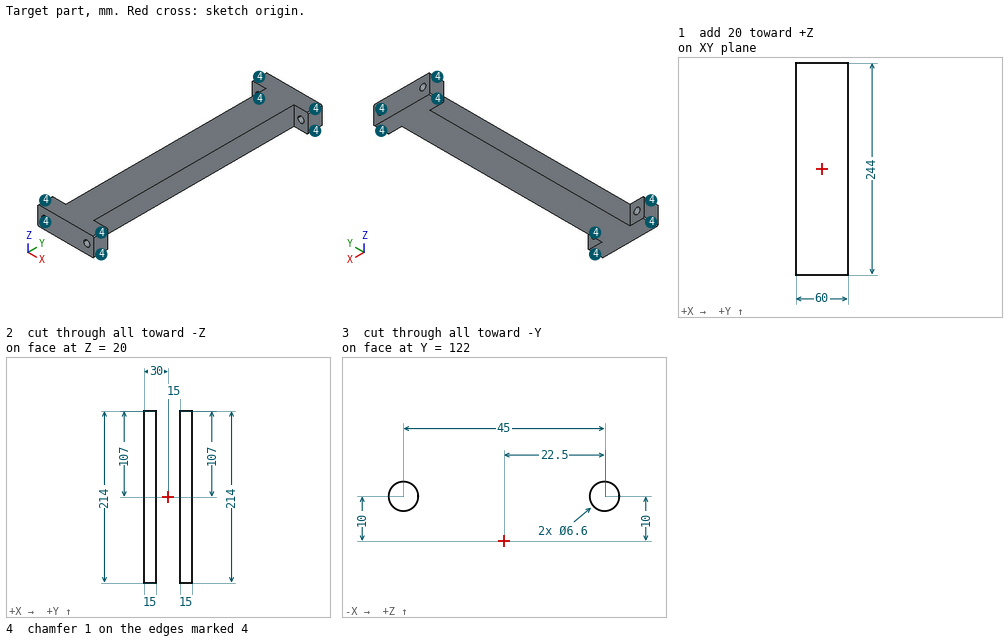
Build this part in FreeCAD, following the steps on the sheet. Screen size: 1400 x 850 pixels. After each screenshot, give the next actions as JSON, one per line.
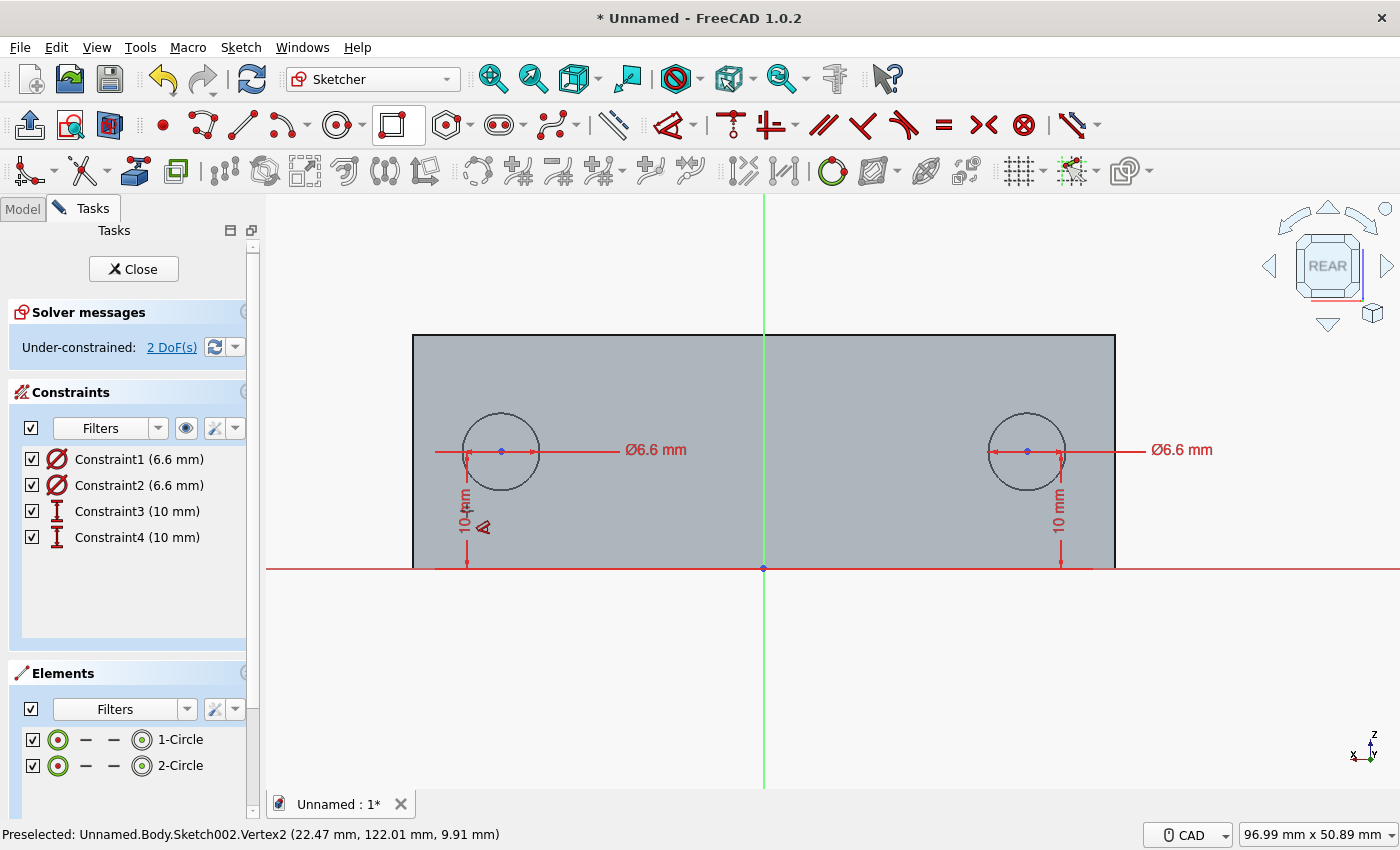
{"action": "left_click", "coordinate": [1027, 452]}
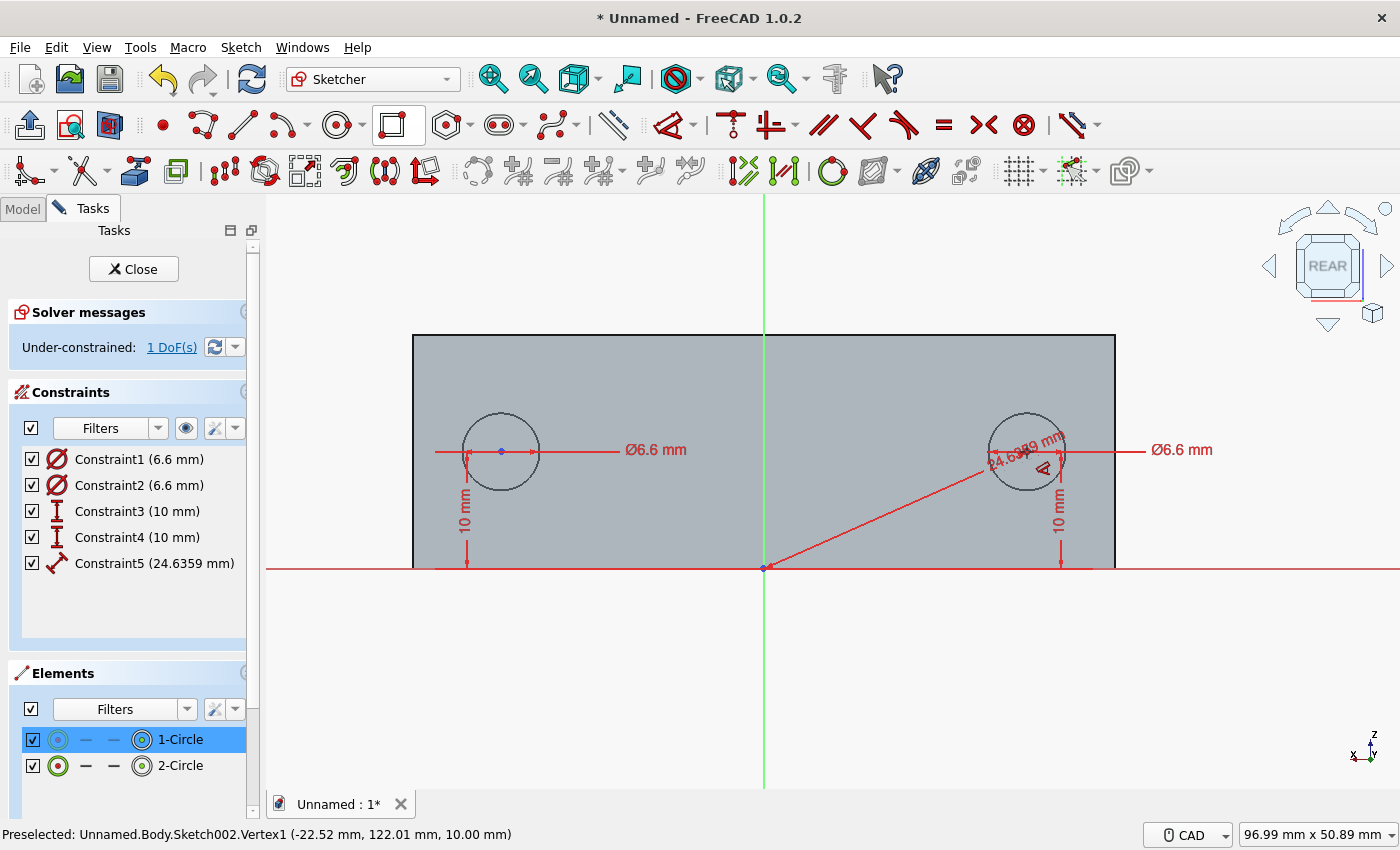
{"action": "left_click", "coordinate": [501, 452]}
{"action": "left_click", "coordinate": [643, 418]}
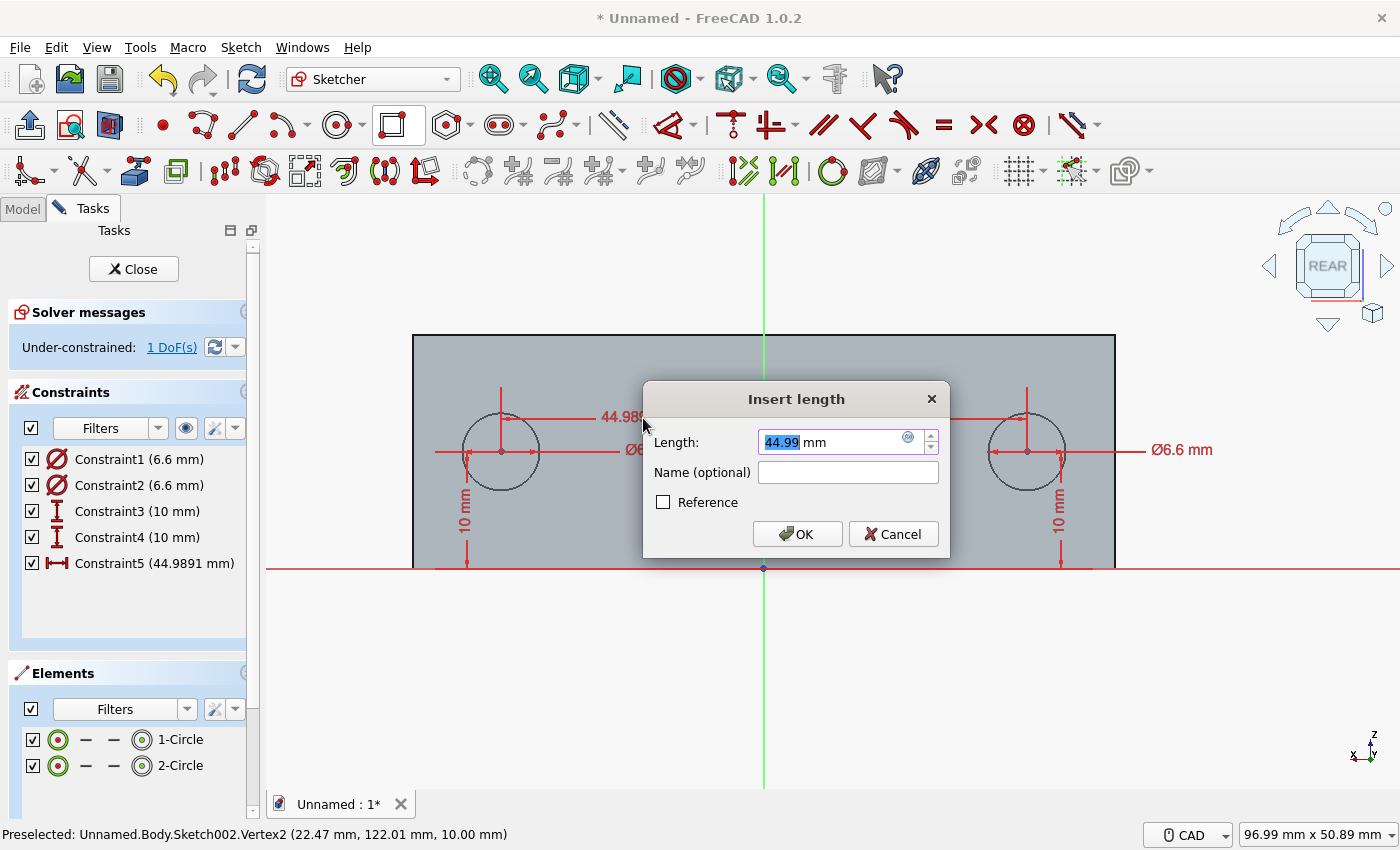
{"action": "type", "text": "45"}
{"action": "key", "text": "Return"}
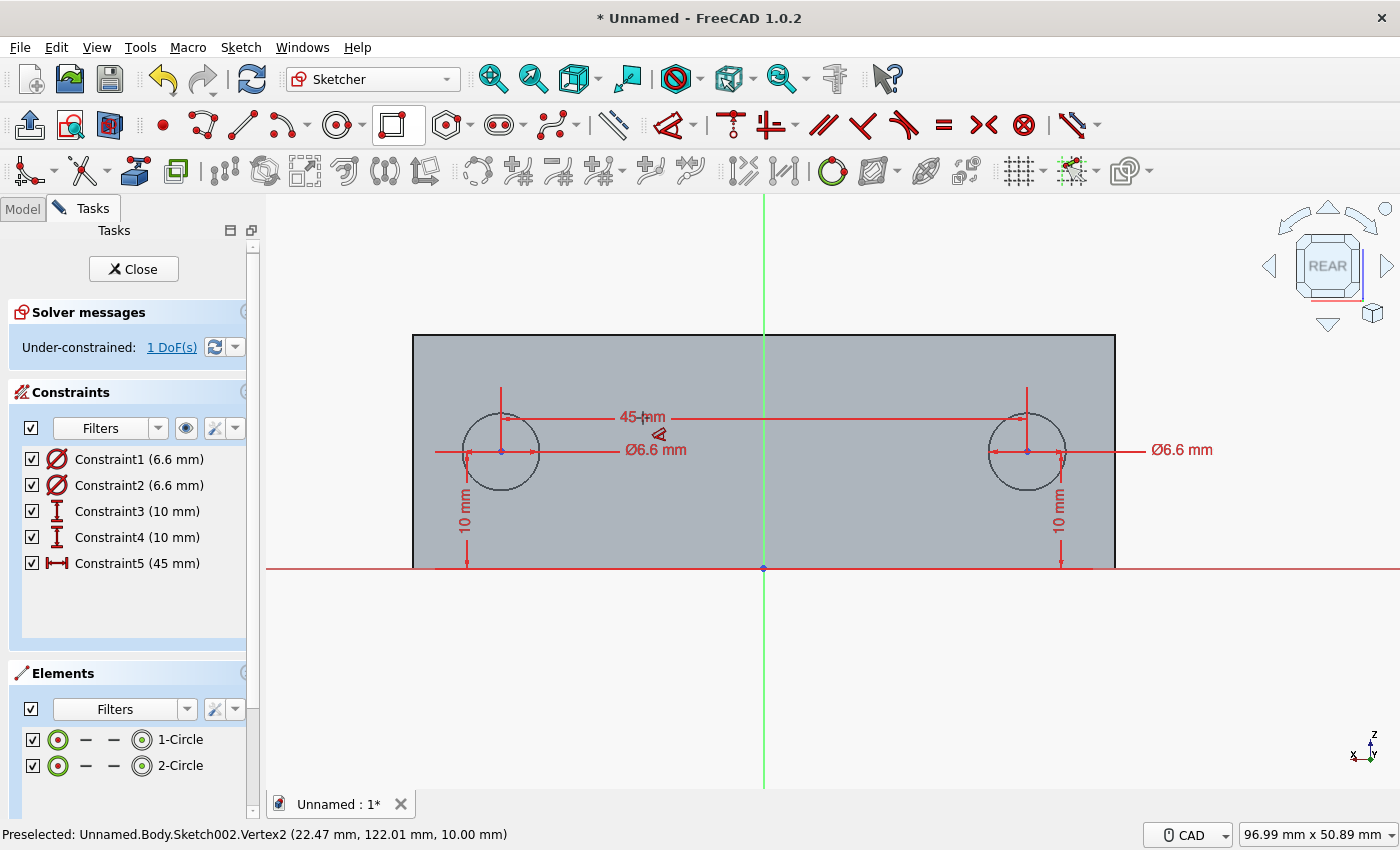
{"action": "left_click", "coordinate": [1027, 452]}
{"action": "left_click", "coordinate": [895, 603]}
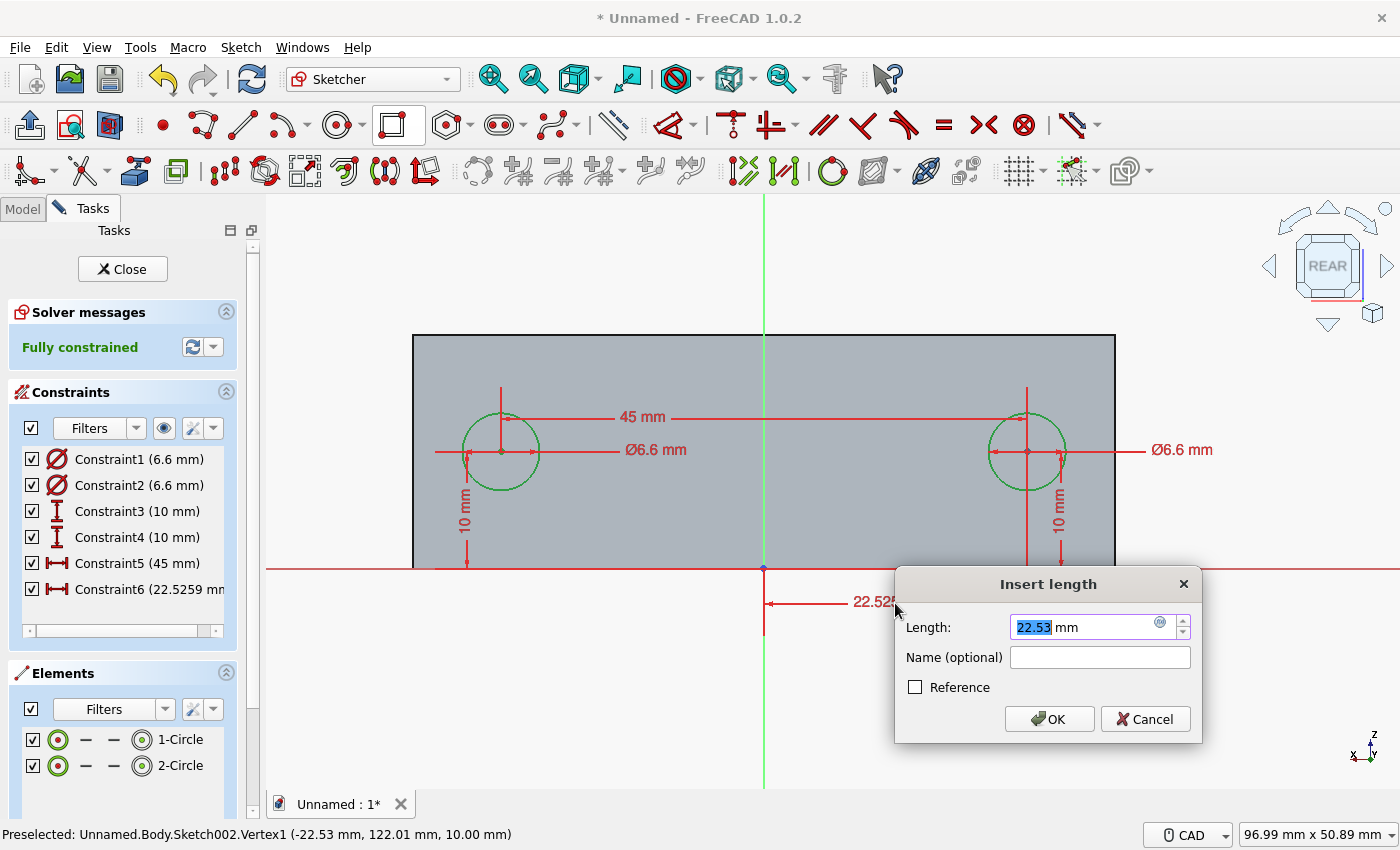
{"action": "type", "text": "22.5"}
{"action": "key", "text": "Return"}
{"action": "key", "text": "Escape"}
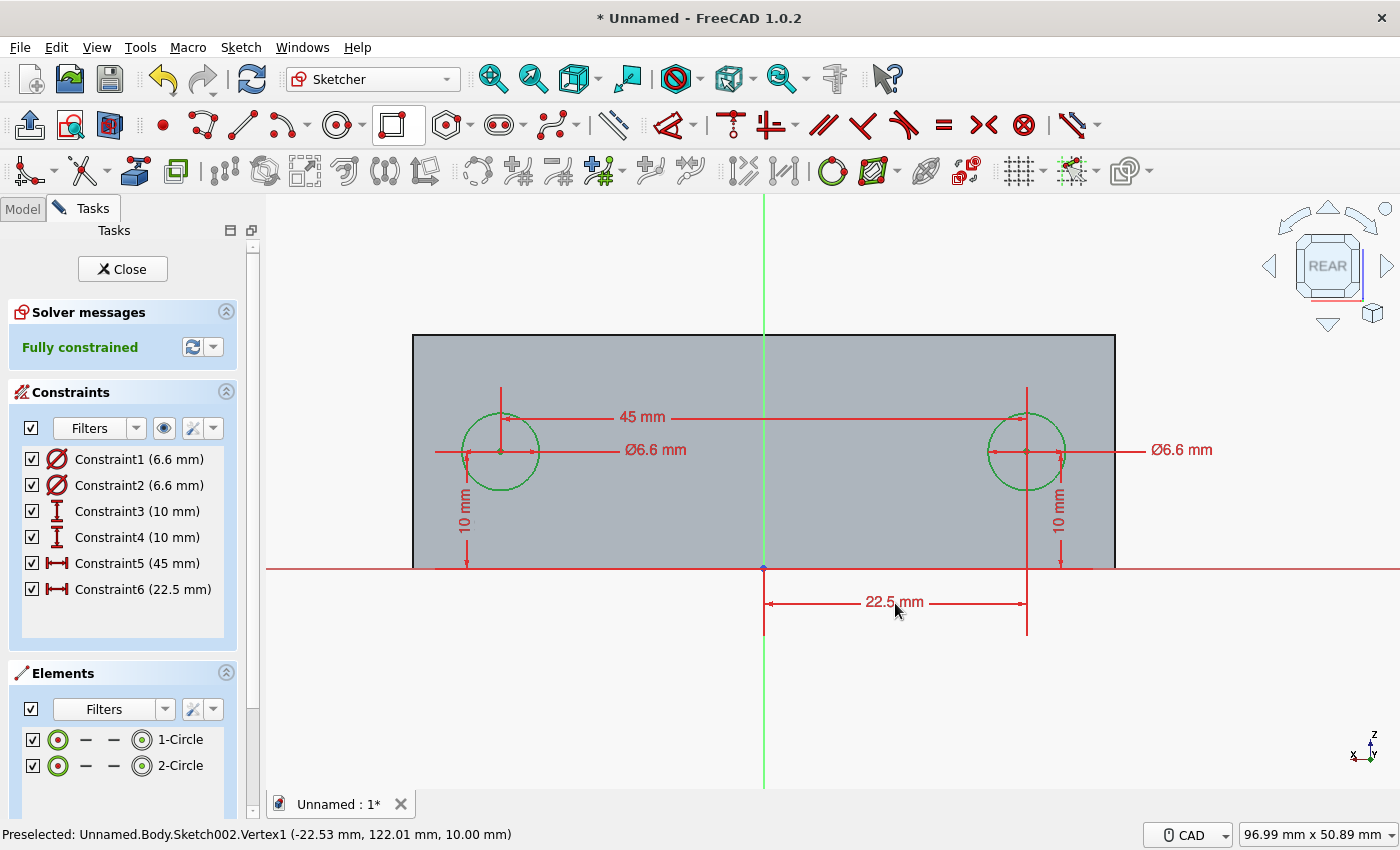
{"action": "left_click", "coordinate": [123, 269]}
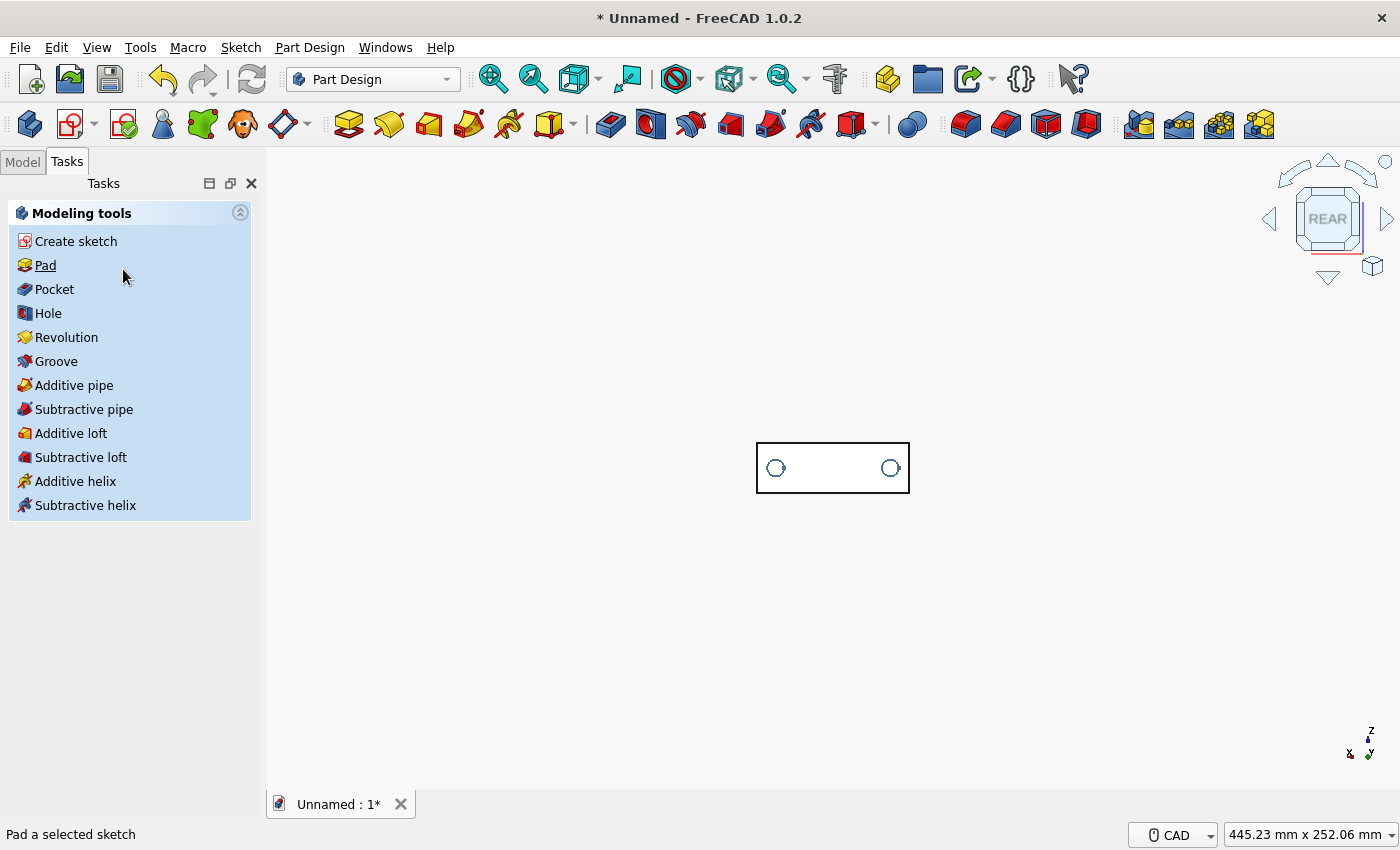
{"action": "left_click", "coordinate": [612, 124]}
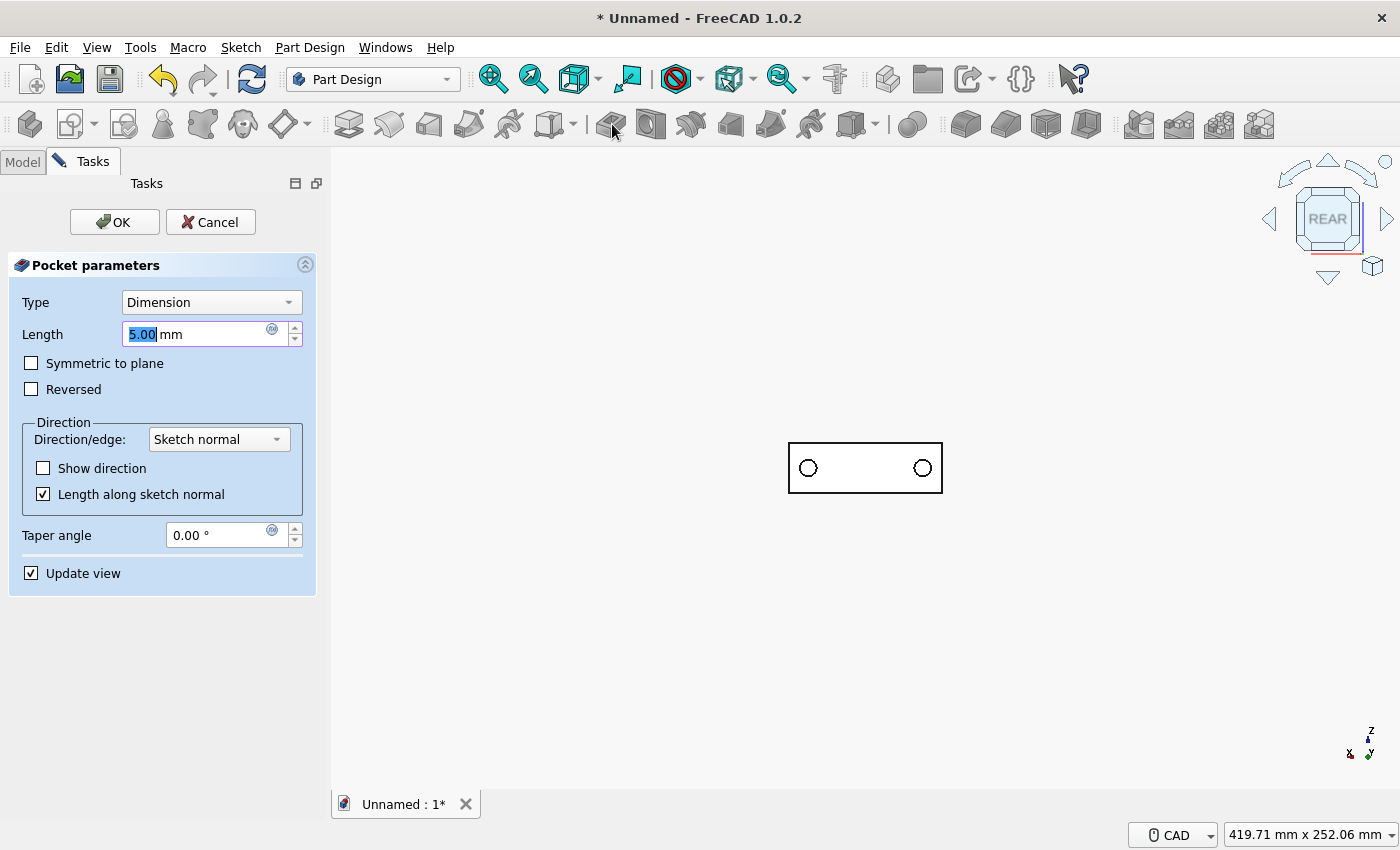
{"action": "left_click", "coordinate": [212, 302]}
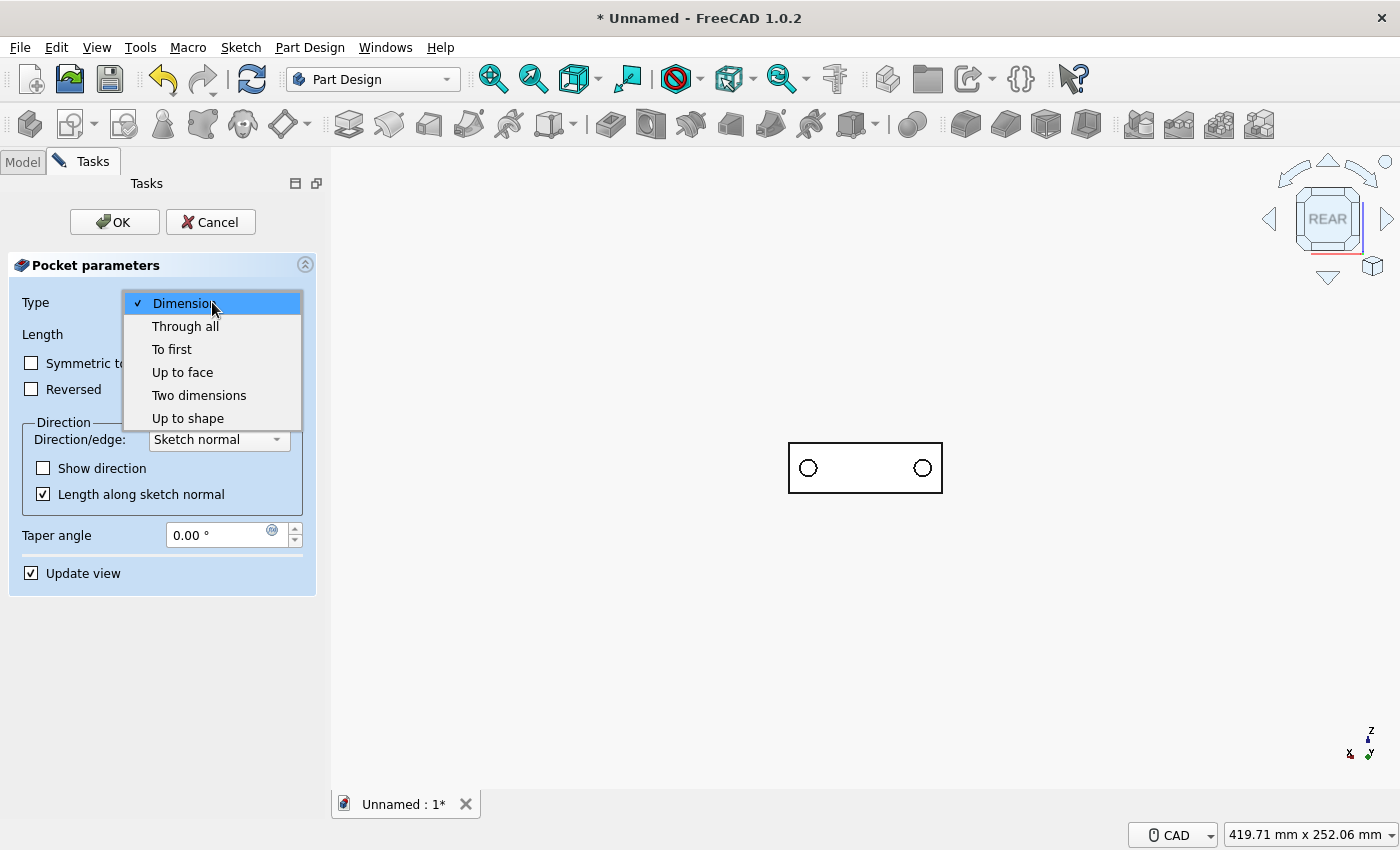
{"action": "left_click", "coordinate": [212, 326]}